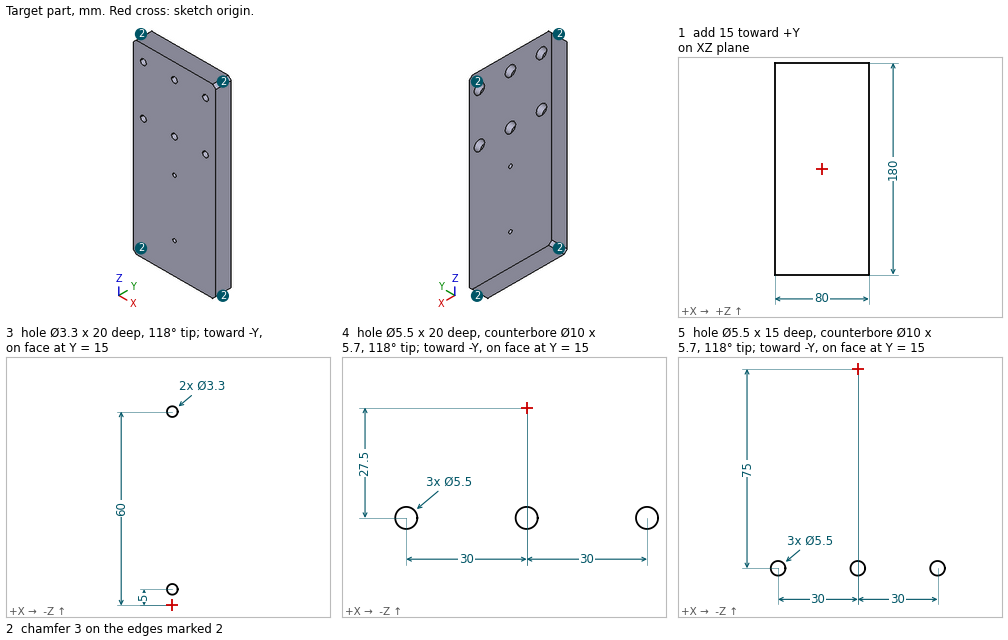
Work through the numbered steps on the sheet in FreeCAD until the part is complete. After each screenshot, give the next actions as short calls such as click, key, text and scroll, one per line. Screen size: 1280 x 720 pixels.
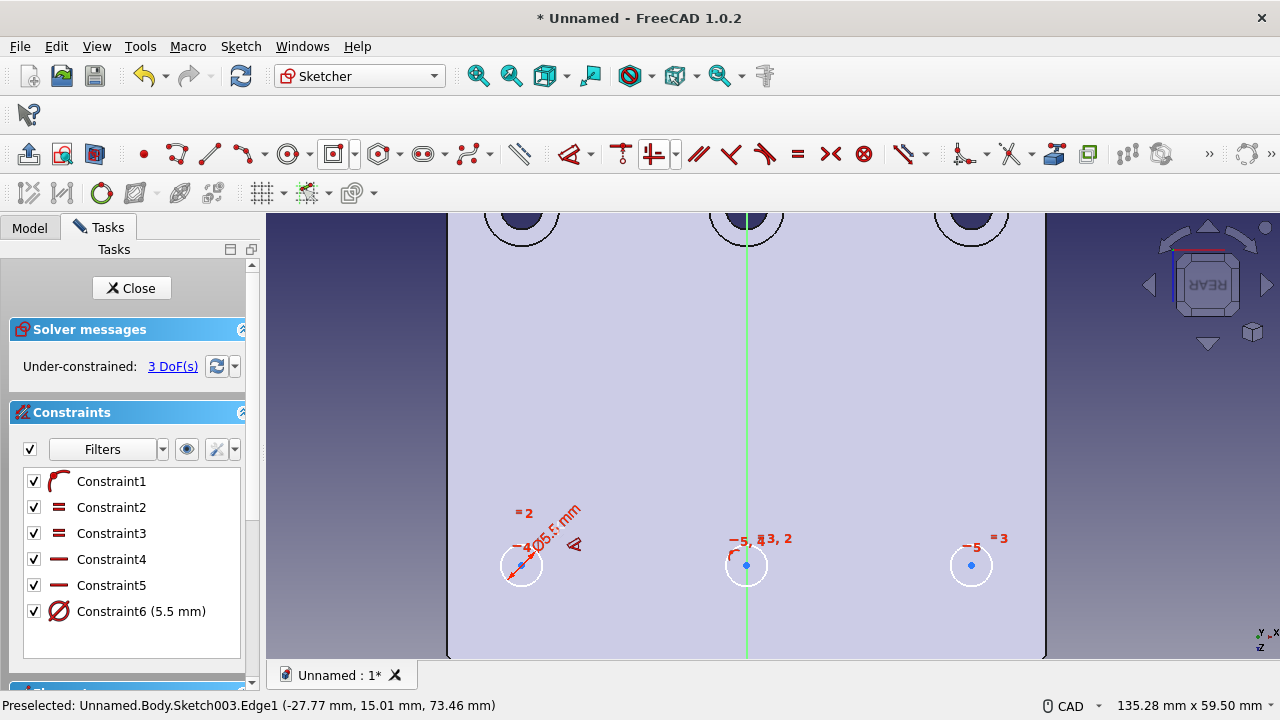
click(522, 566)
click(634, 600)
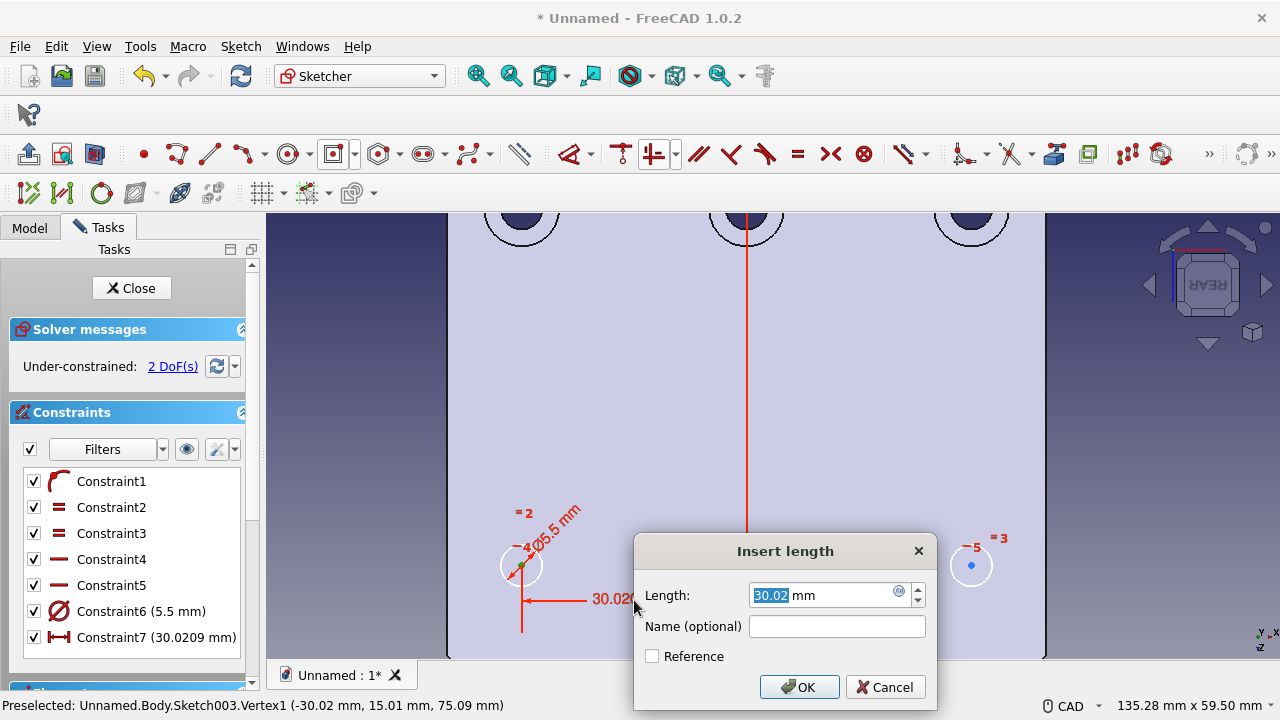
text(30)
key(Return)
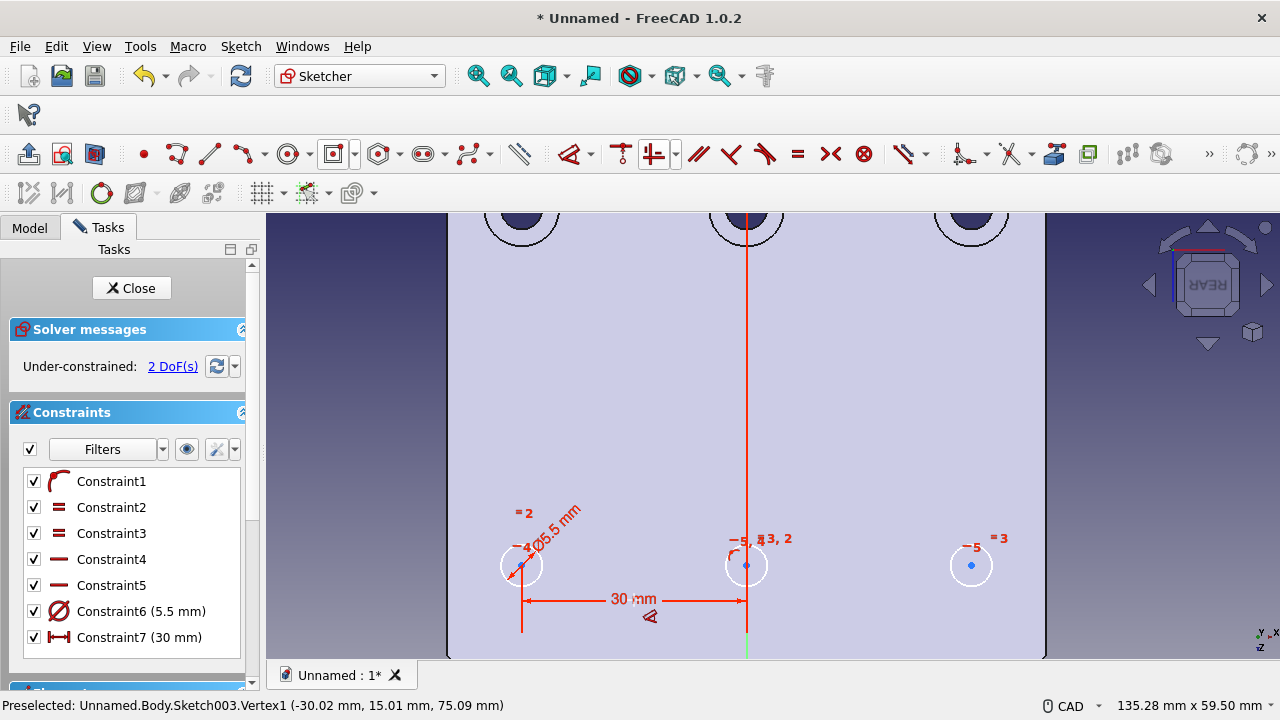
click(522, 566)
click(488, 403)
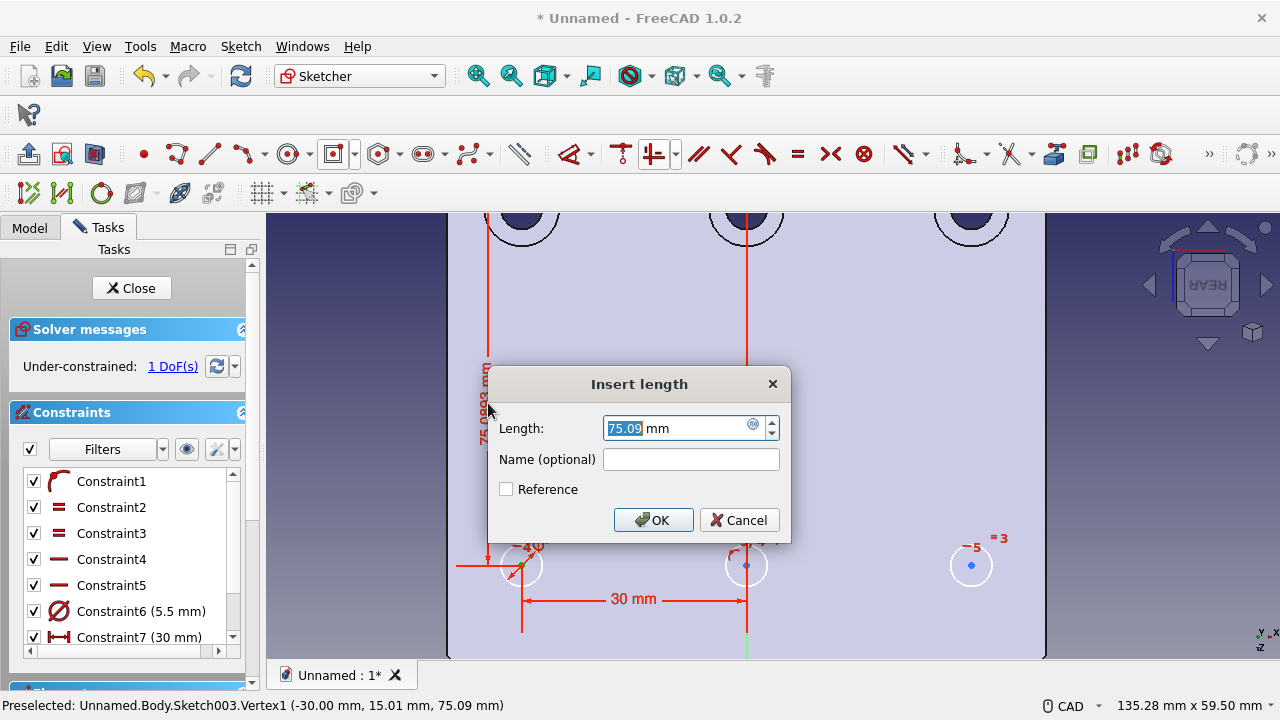
text(75)
key(Return)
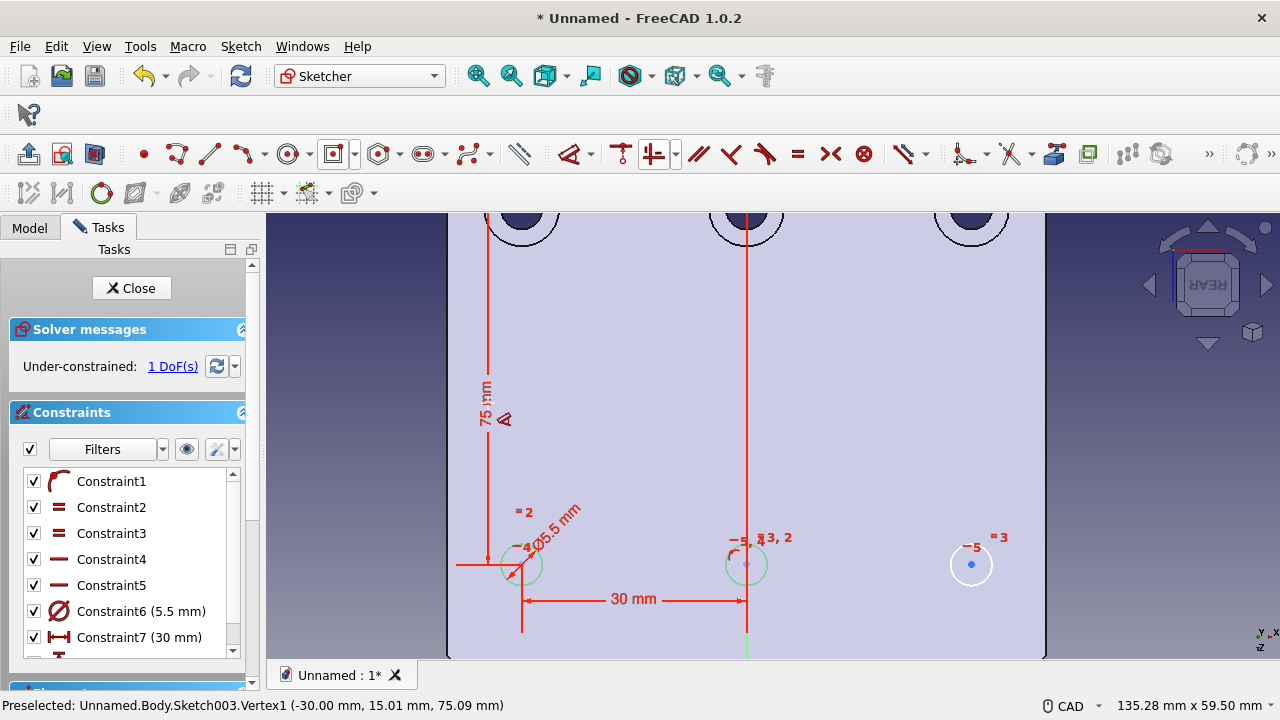
click(971, 565)
click(859, 599)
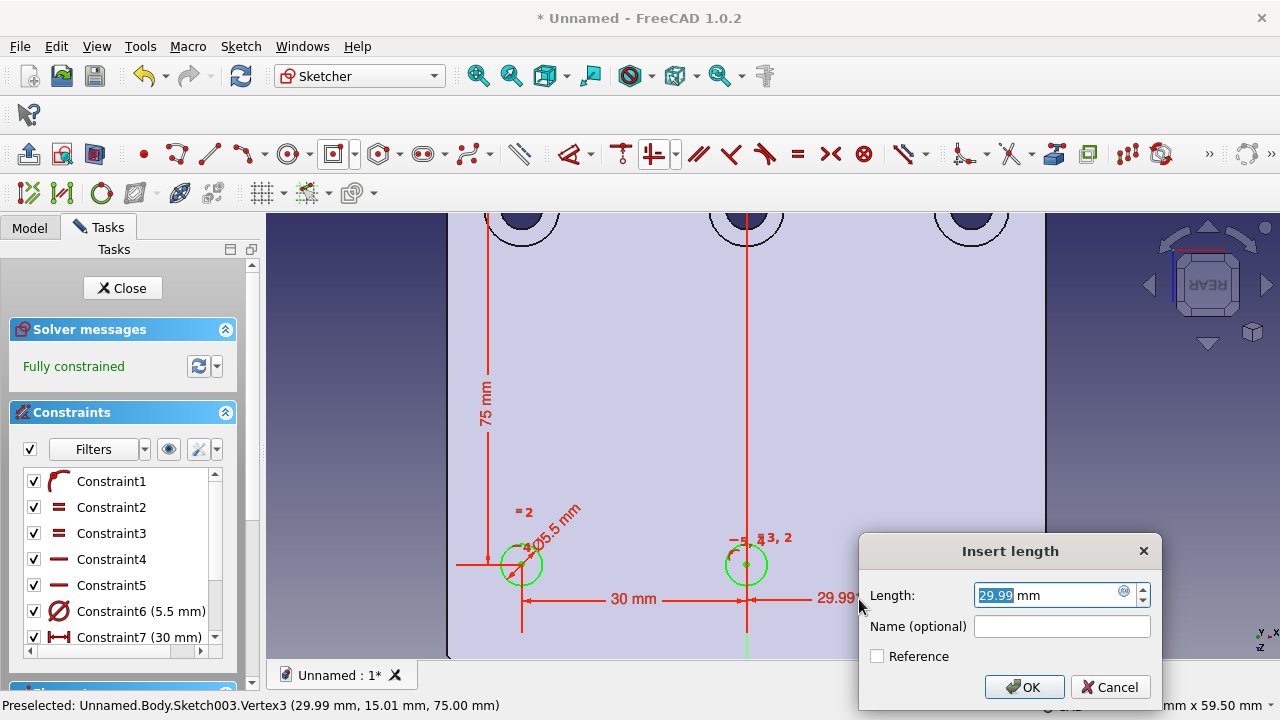
text(30)
key(Return)
key(Escape)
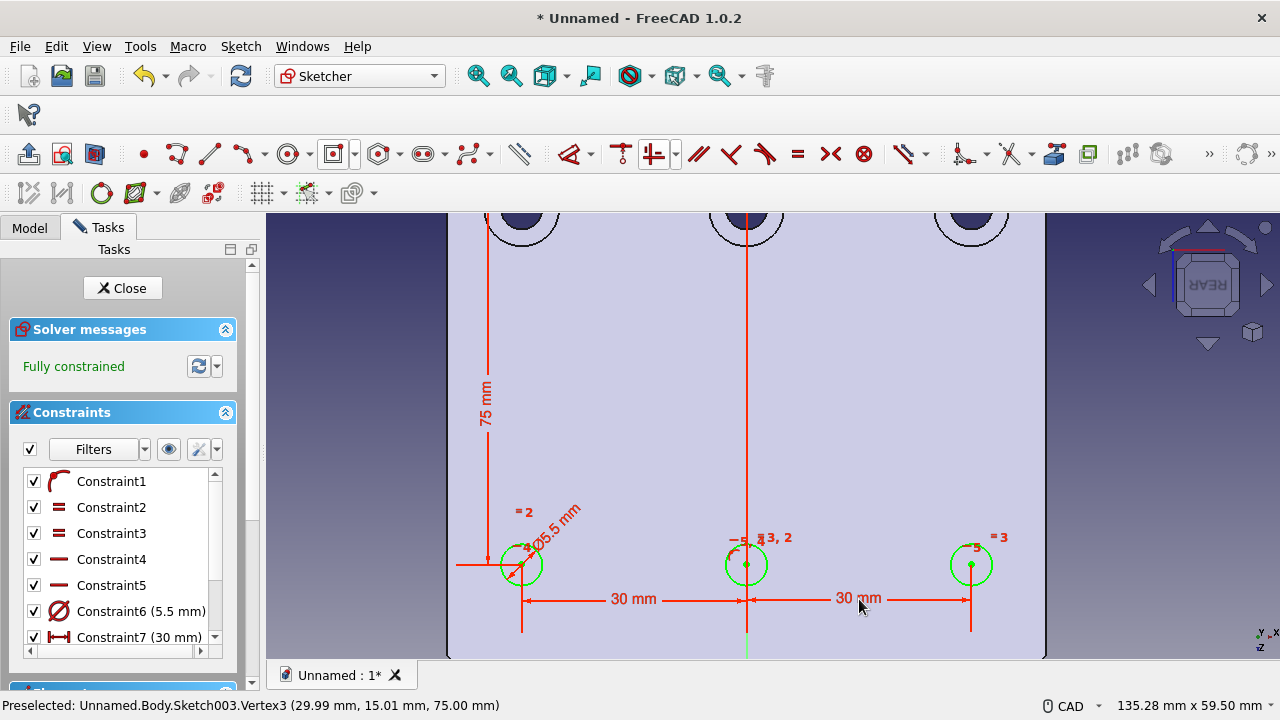
click(123, 288)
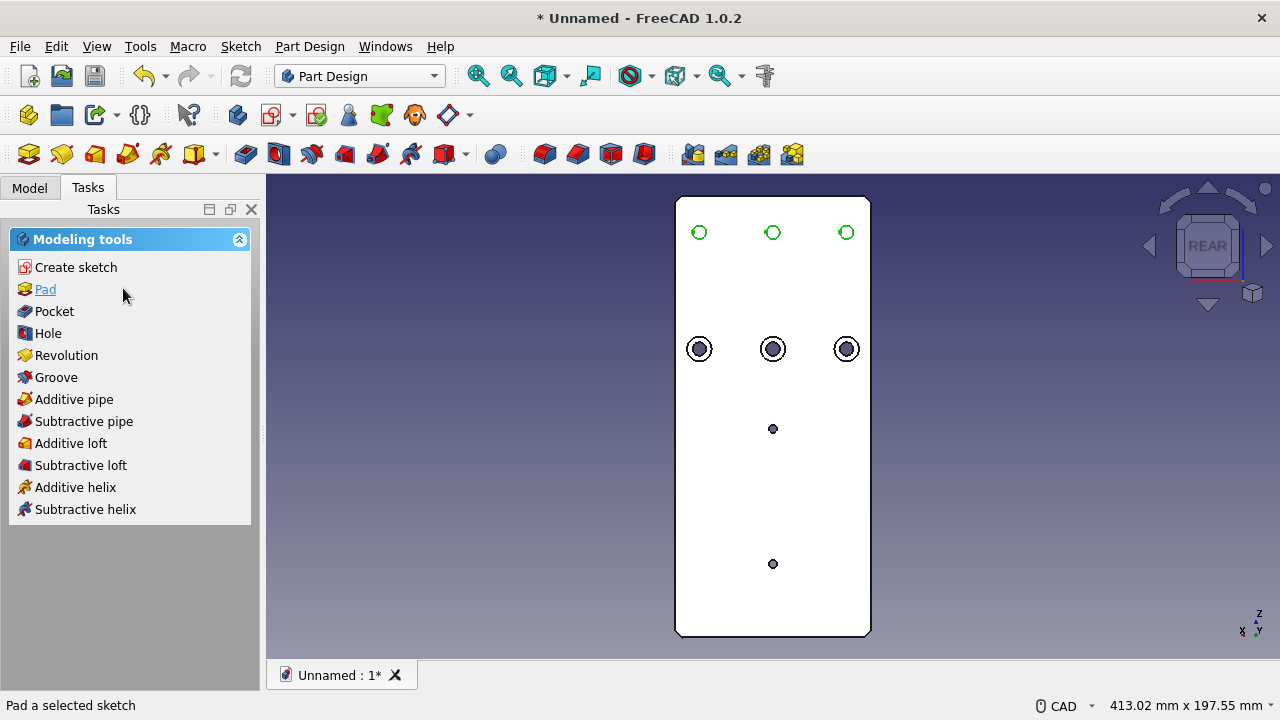
click(279, 154)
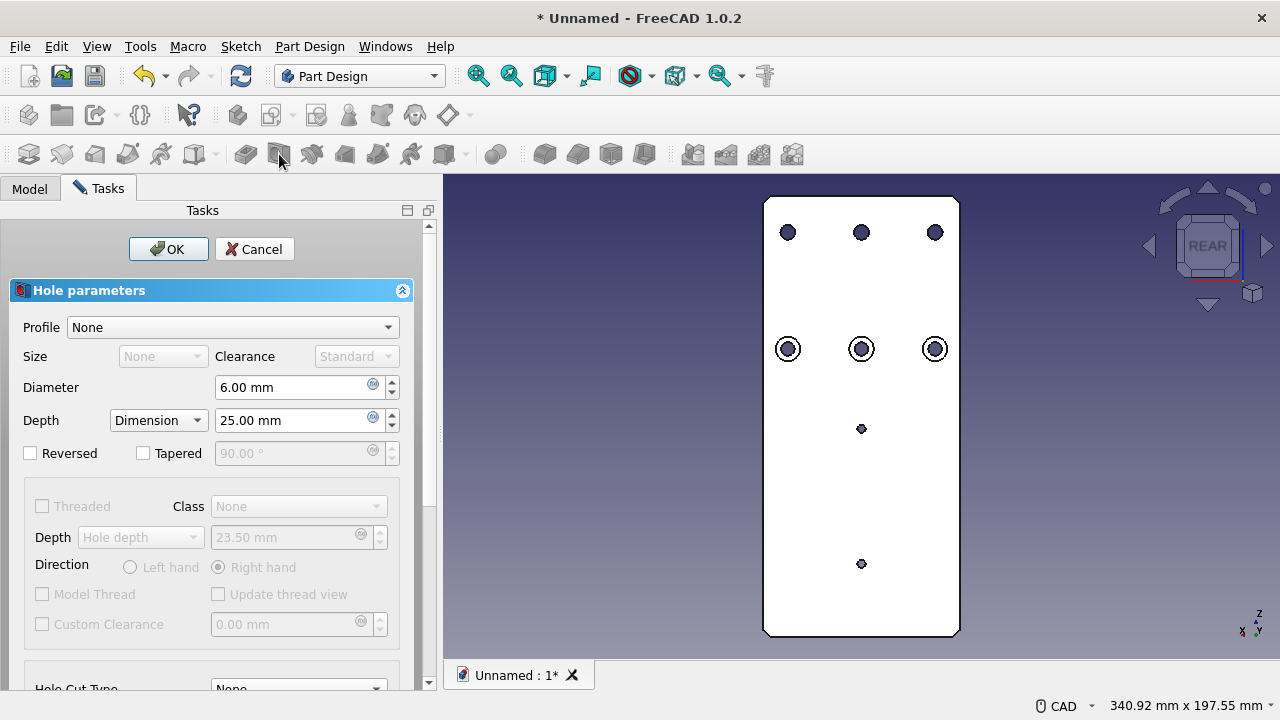
triple_click(300, 388)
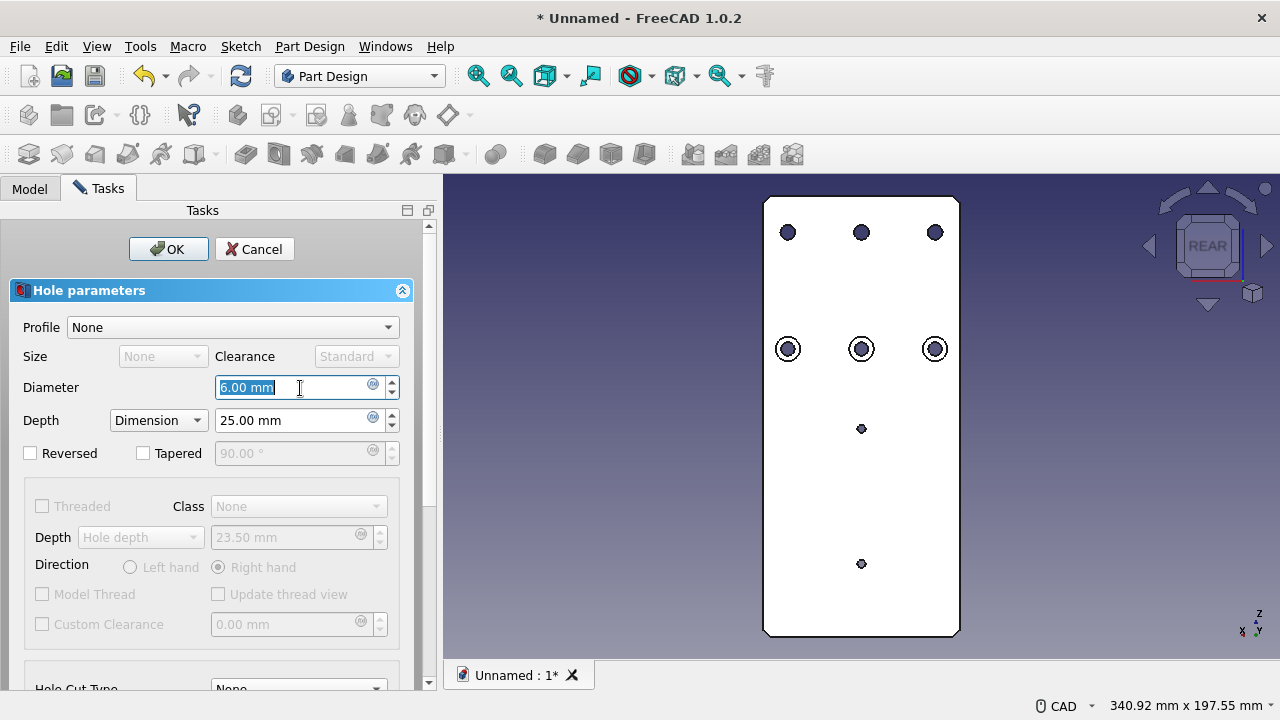
text(5.5)
key(Tab)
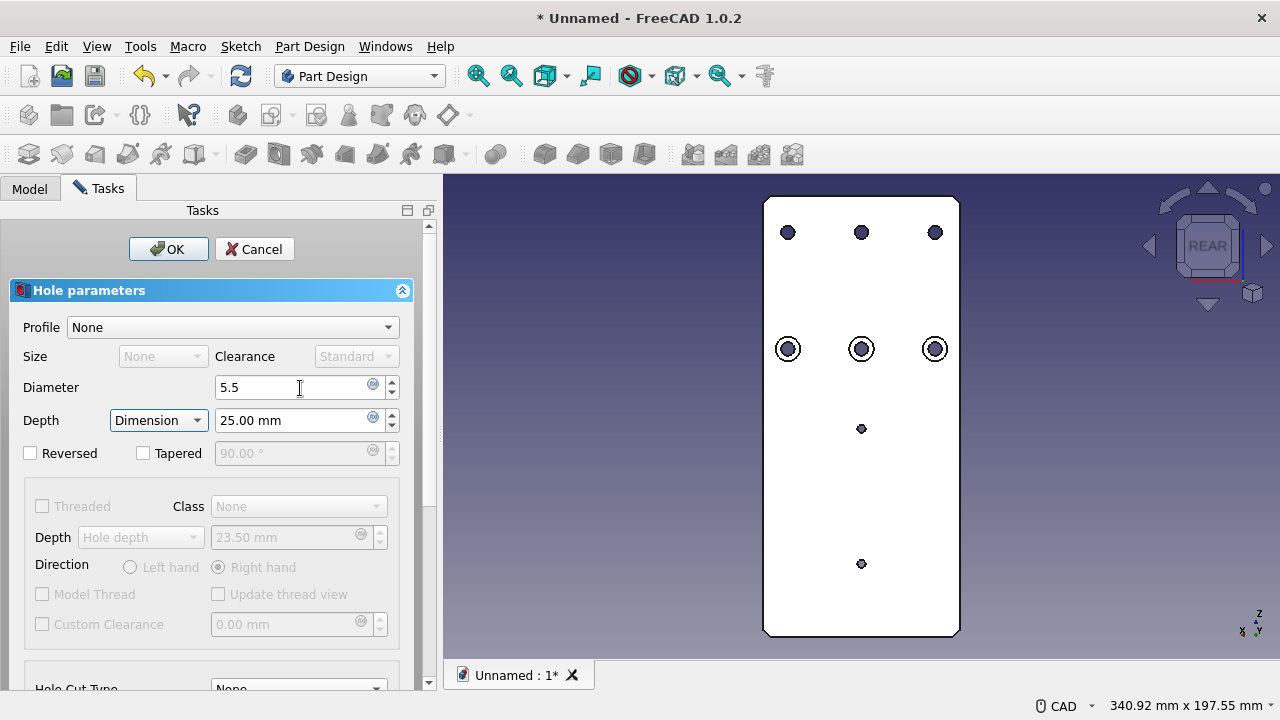
triple_click(300, 420)